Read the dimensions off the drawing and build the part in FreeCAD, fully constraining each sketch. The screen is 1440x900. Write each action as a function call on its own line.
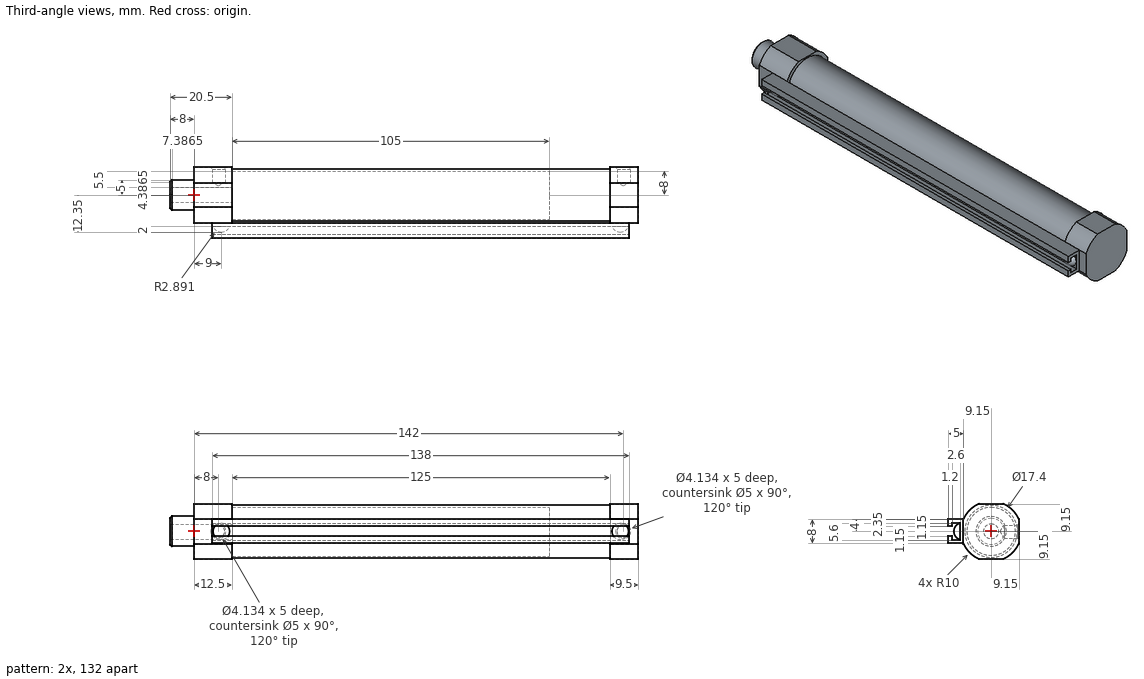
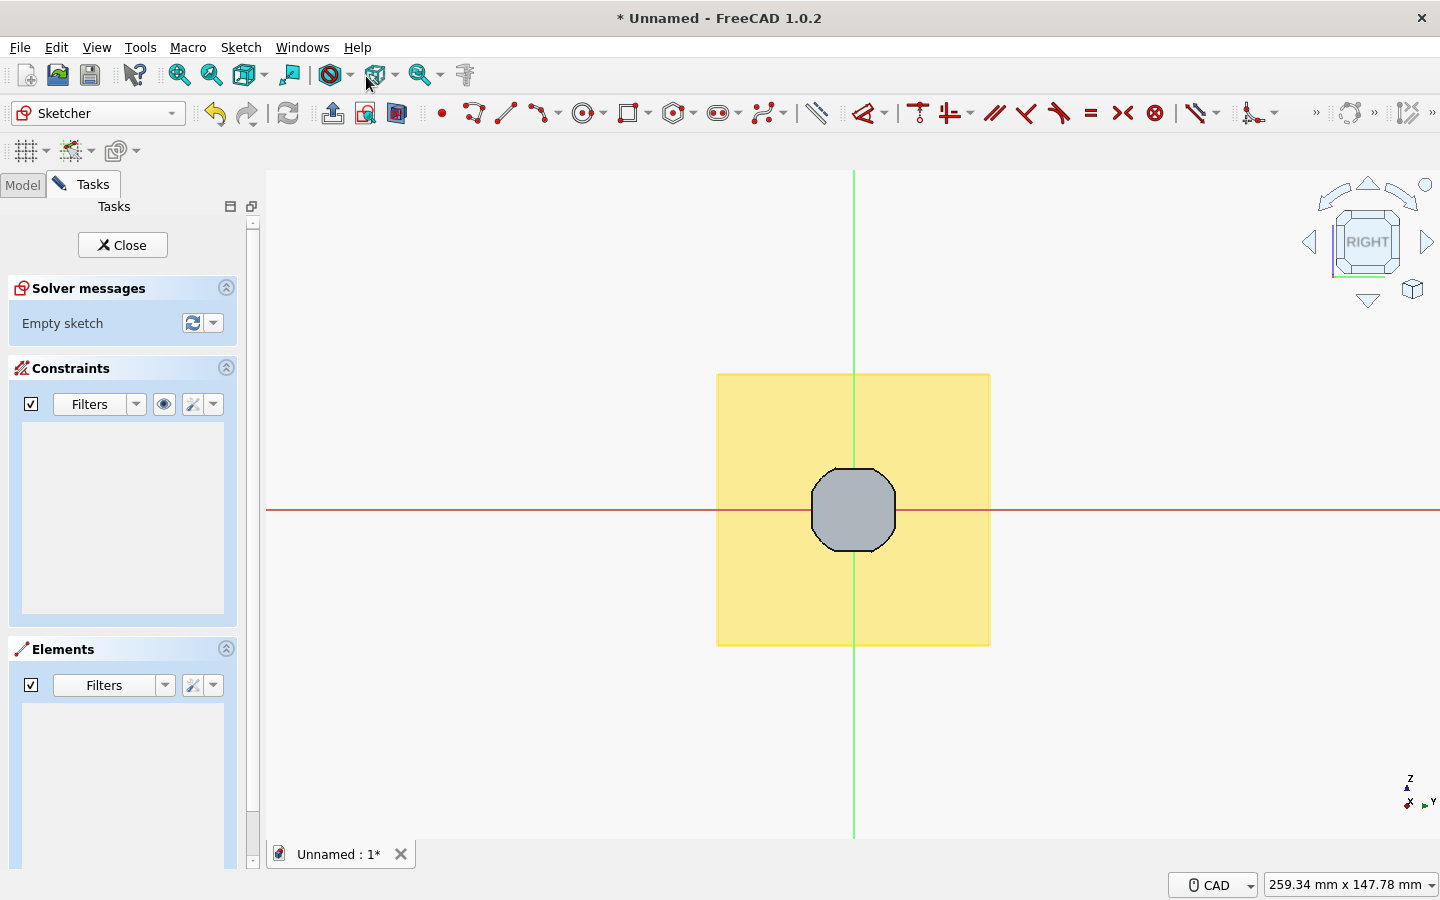
click(398, 114)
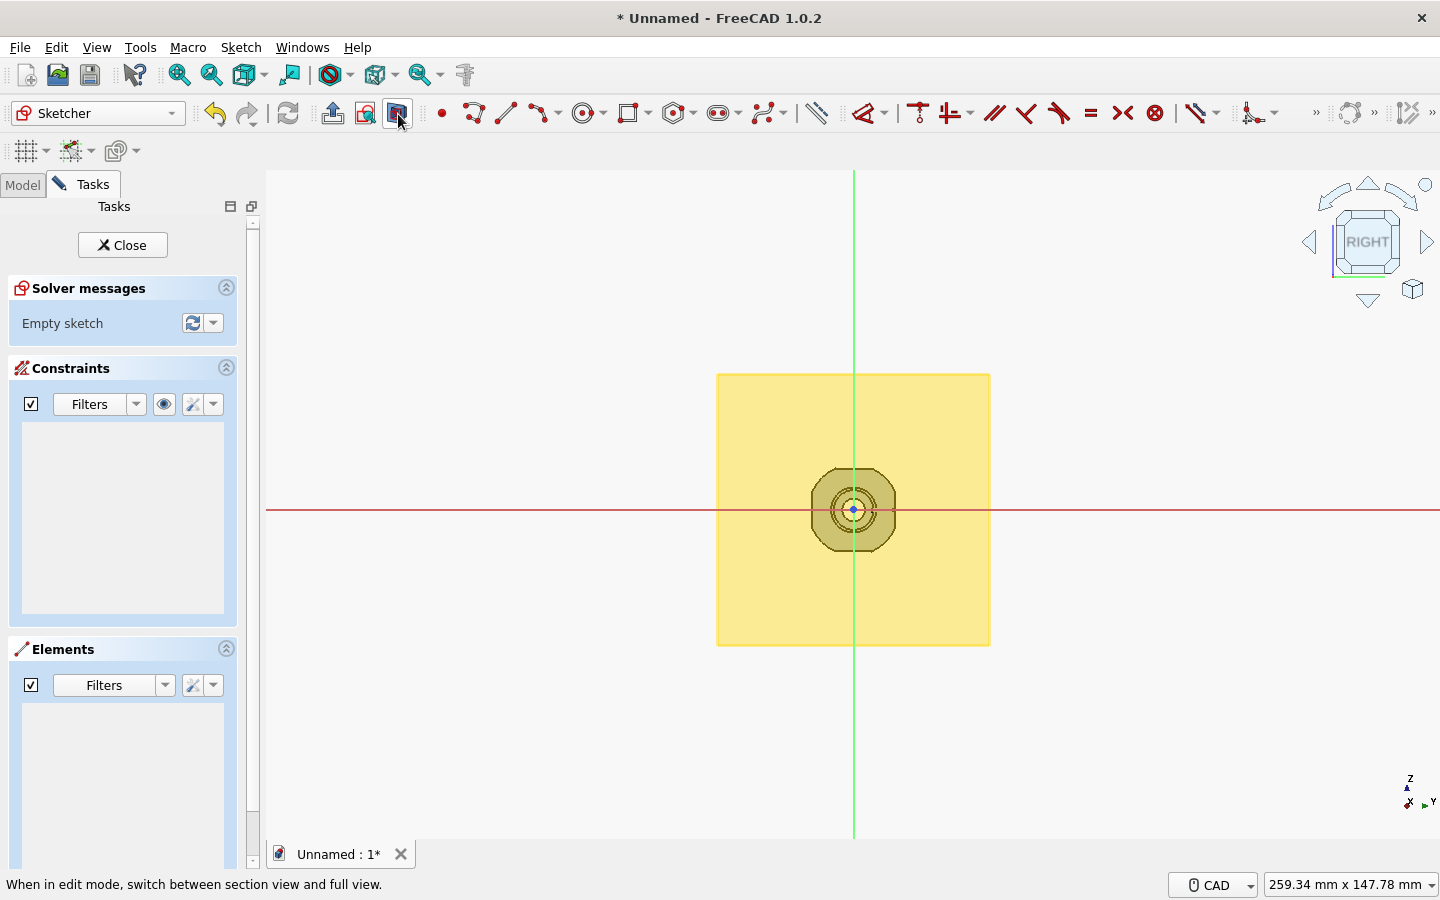
scroll(825, 511, up, 12)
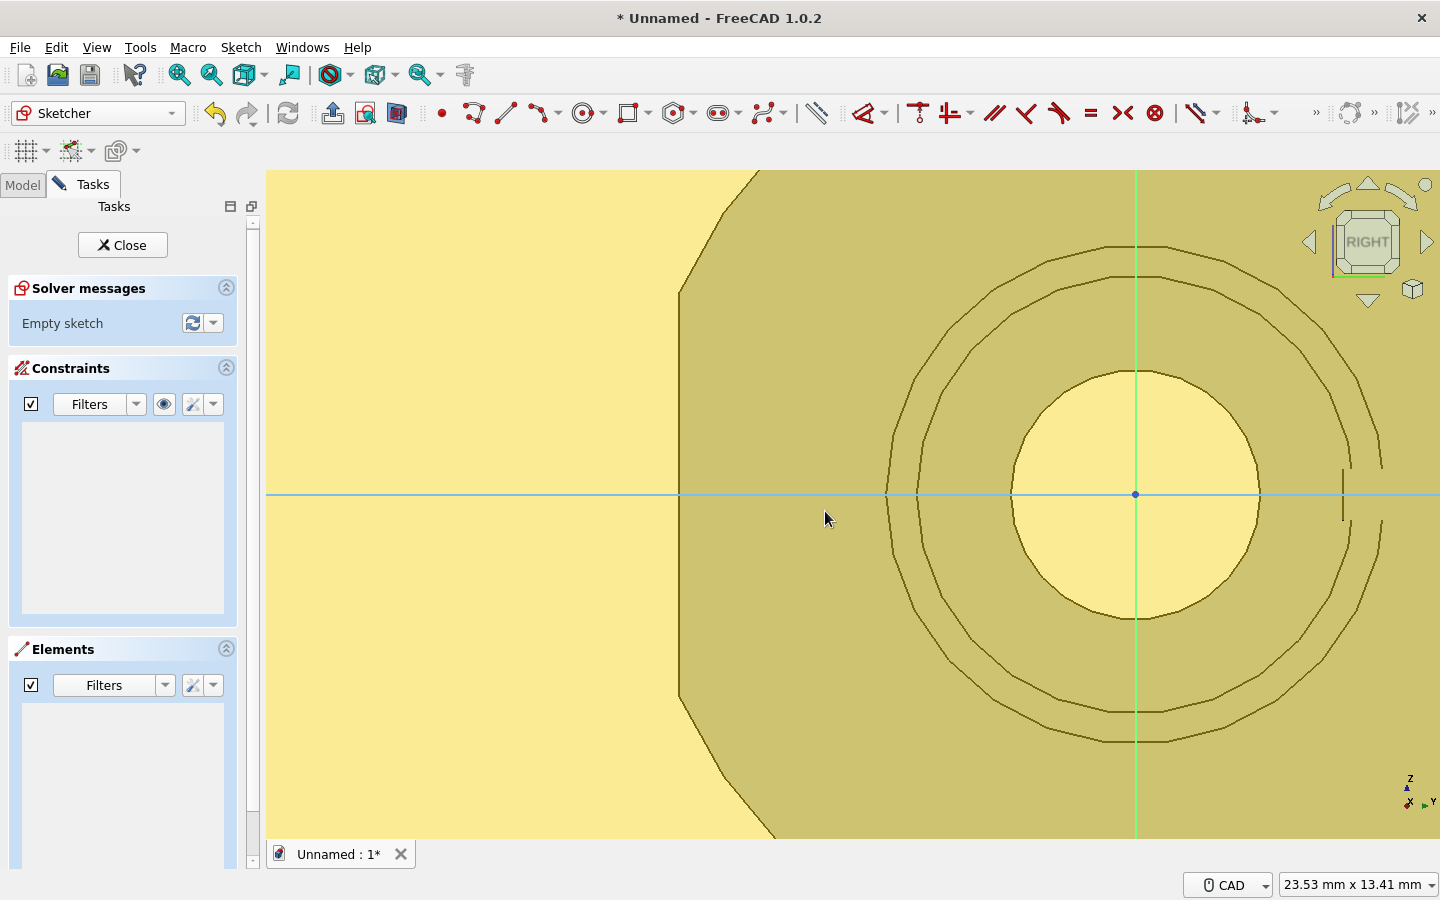
click(474, 114)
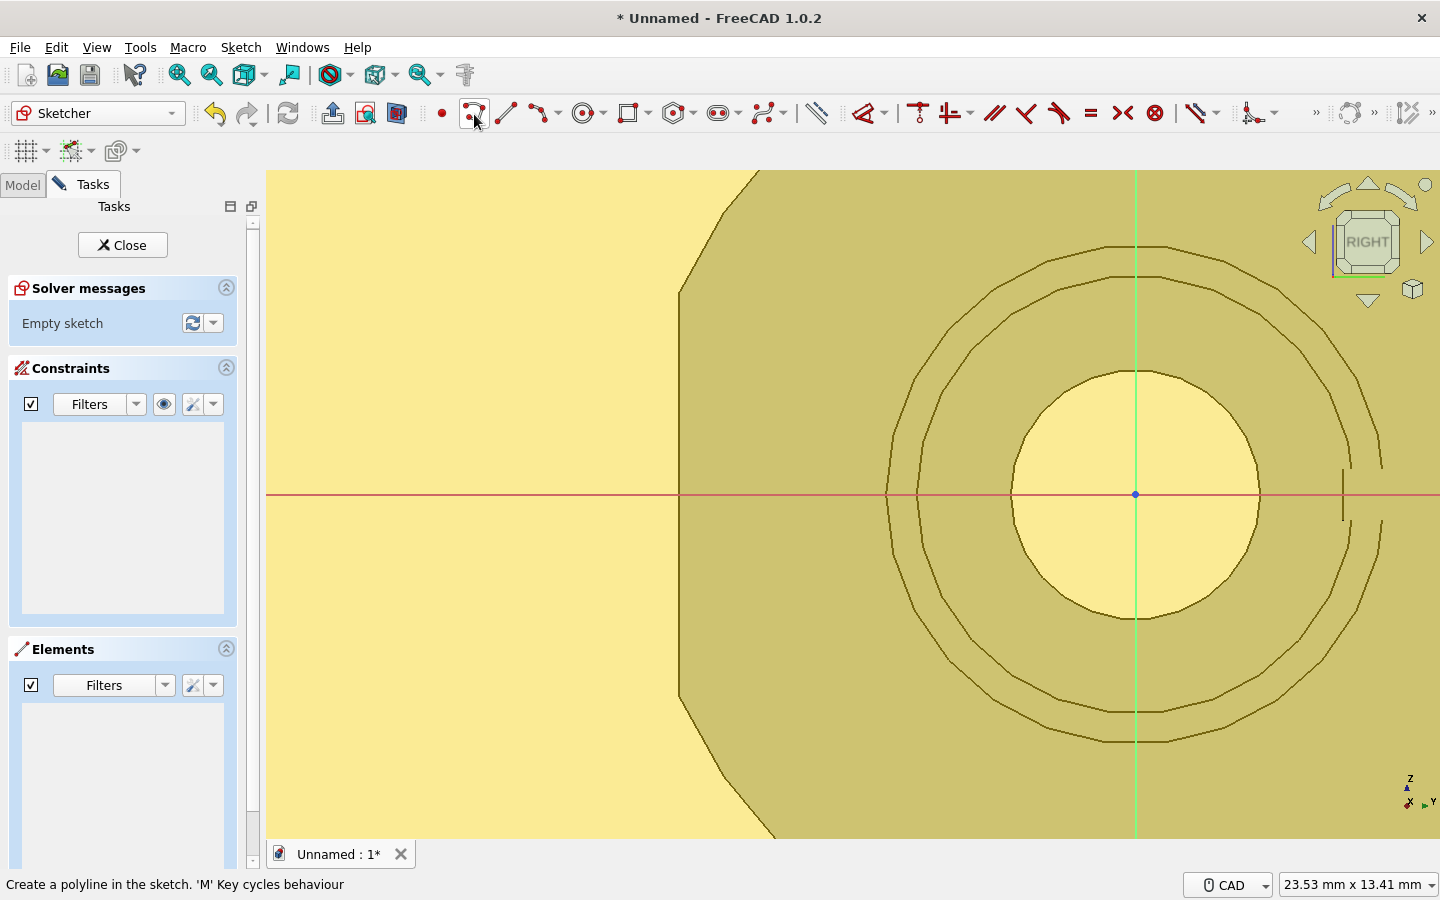
click(679, 295)
click(429, 295)
click(429, 412)
click(489, 412)
click(489, 355)
click(619, 355)
click(619, 634)
click(489, 634)
click(489, 577)
click(429, 577)
click(429, 694)
click(679, 694)
click(679, 296)
key(Escape)
key(Escape)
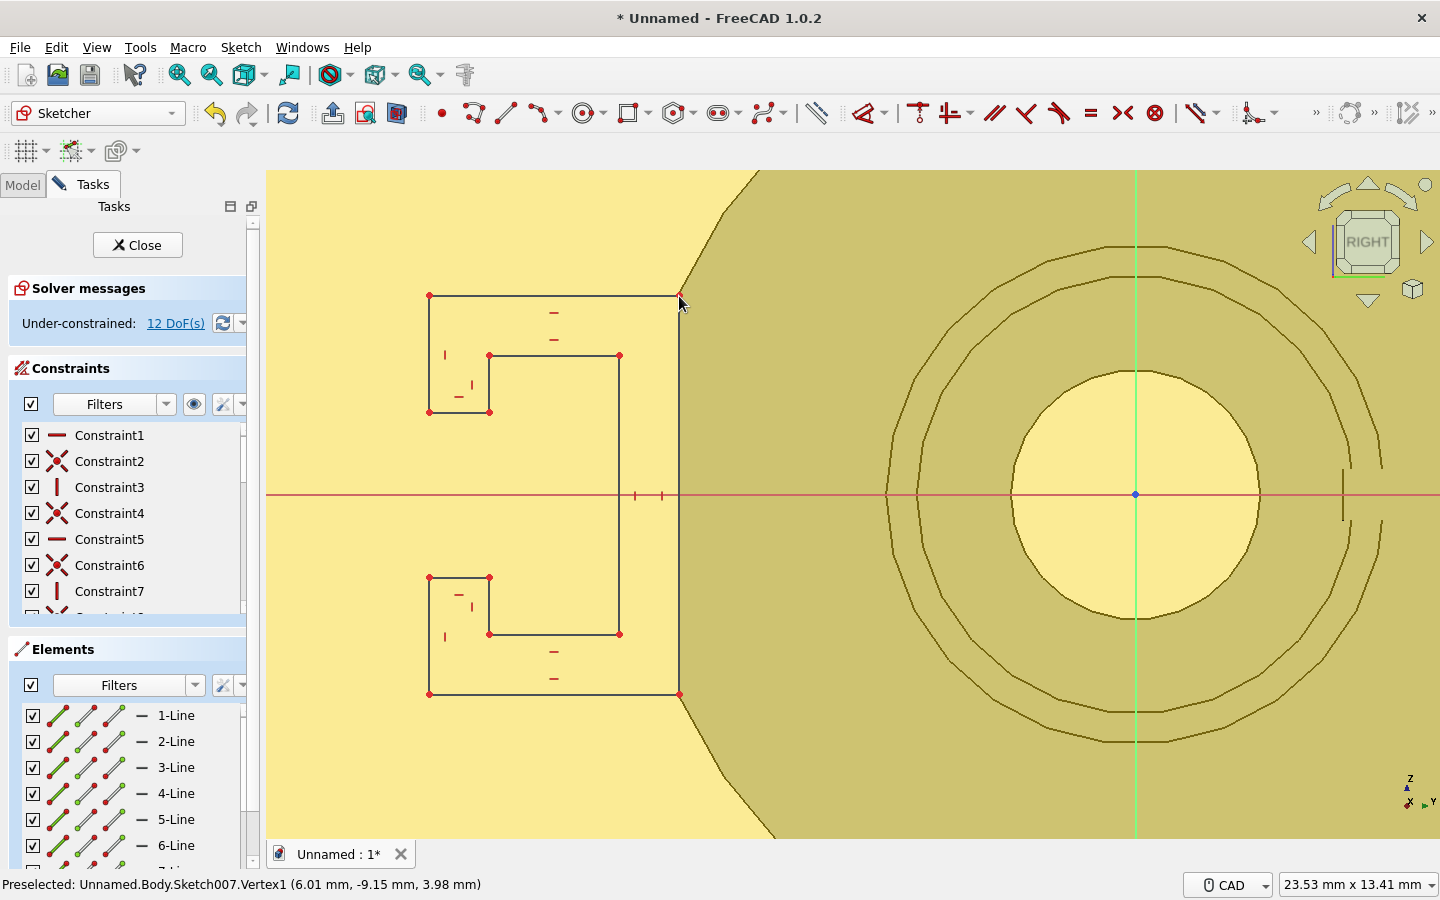
click(864, 114)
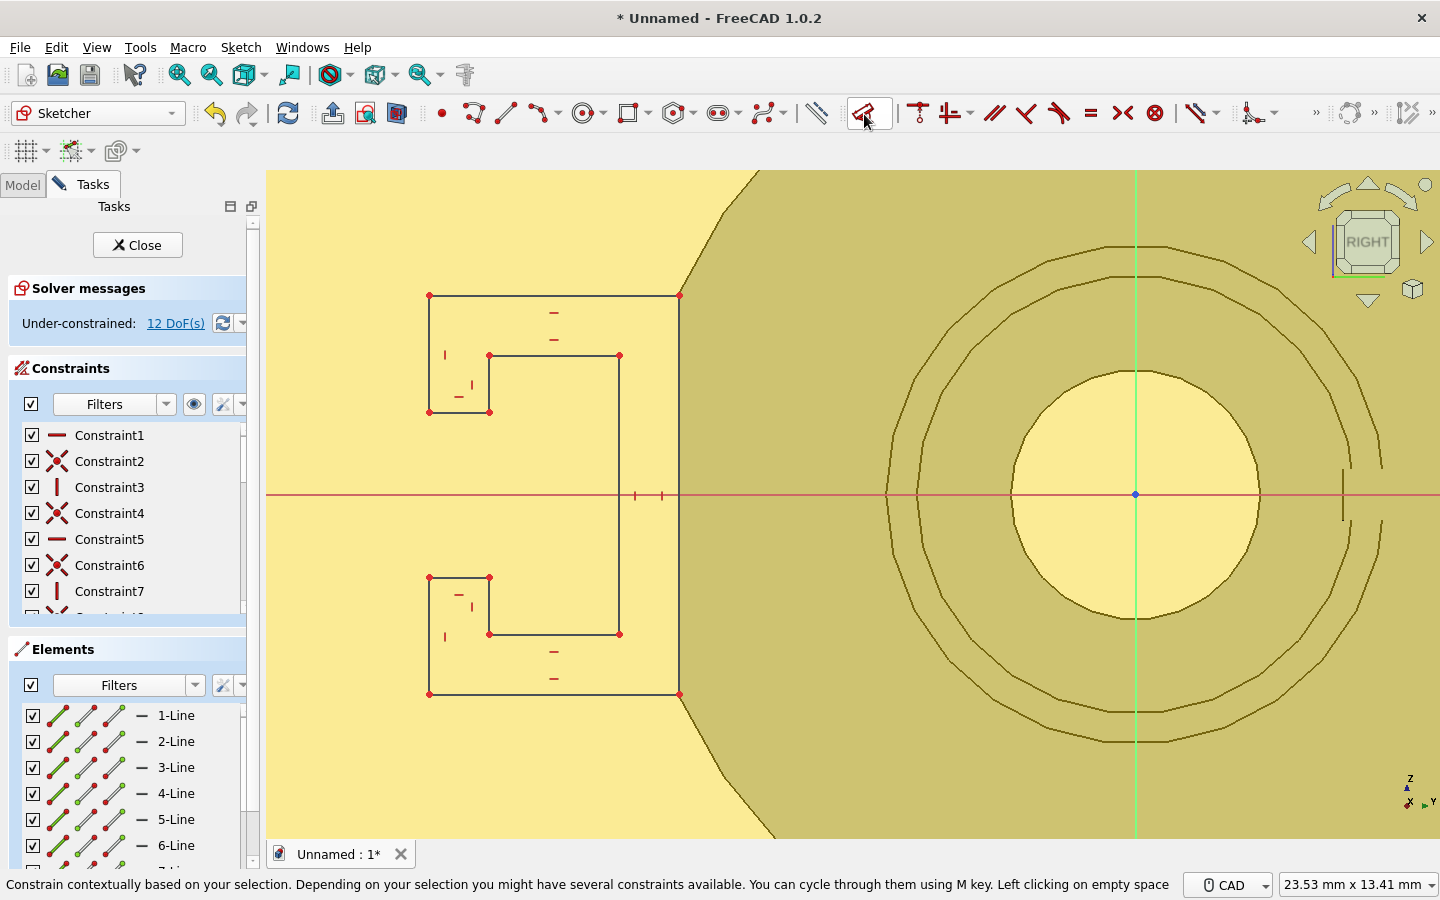
click(604, 296)
click(554, 262)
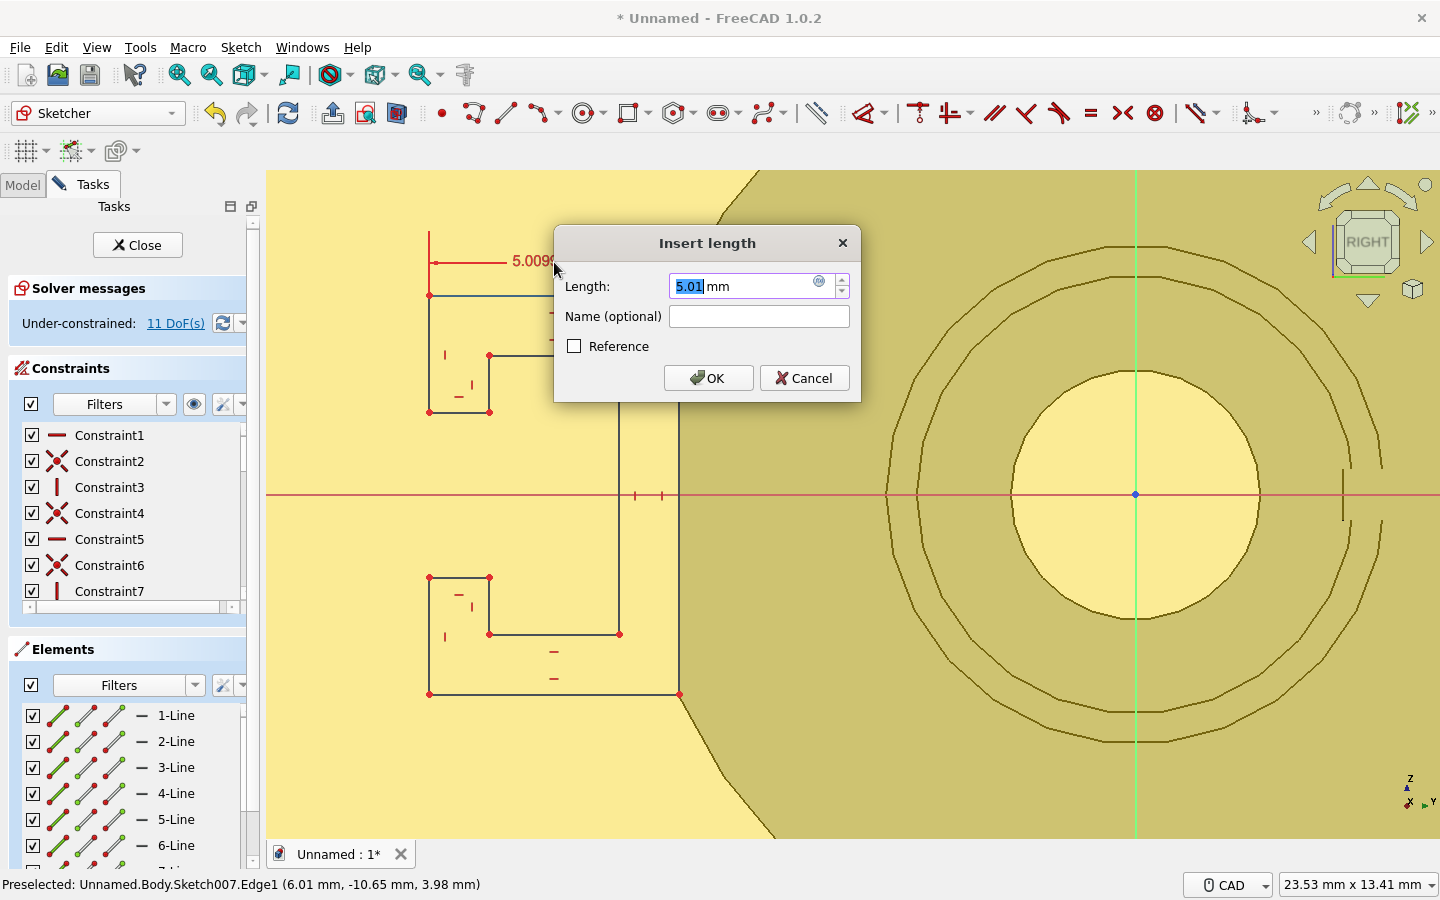
text(5)
key(Return)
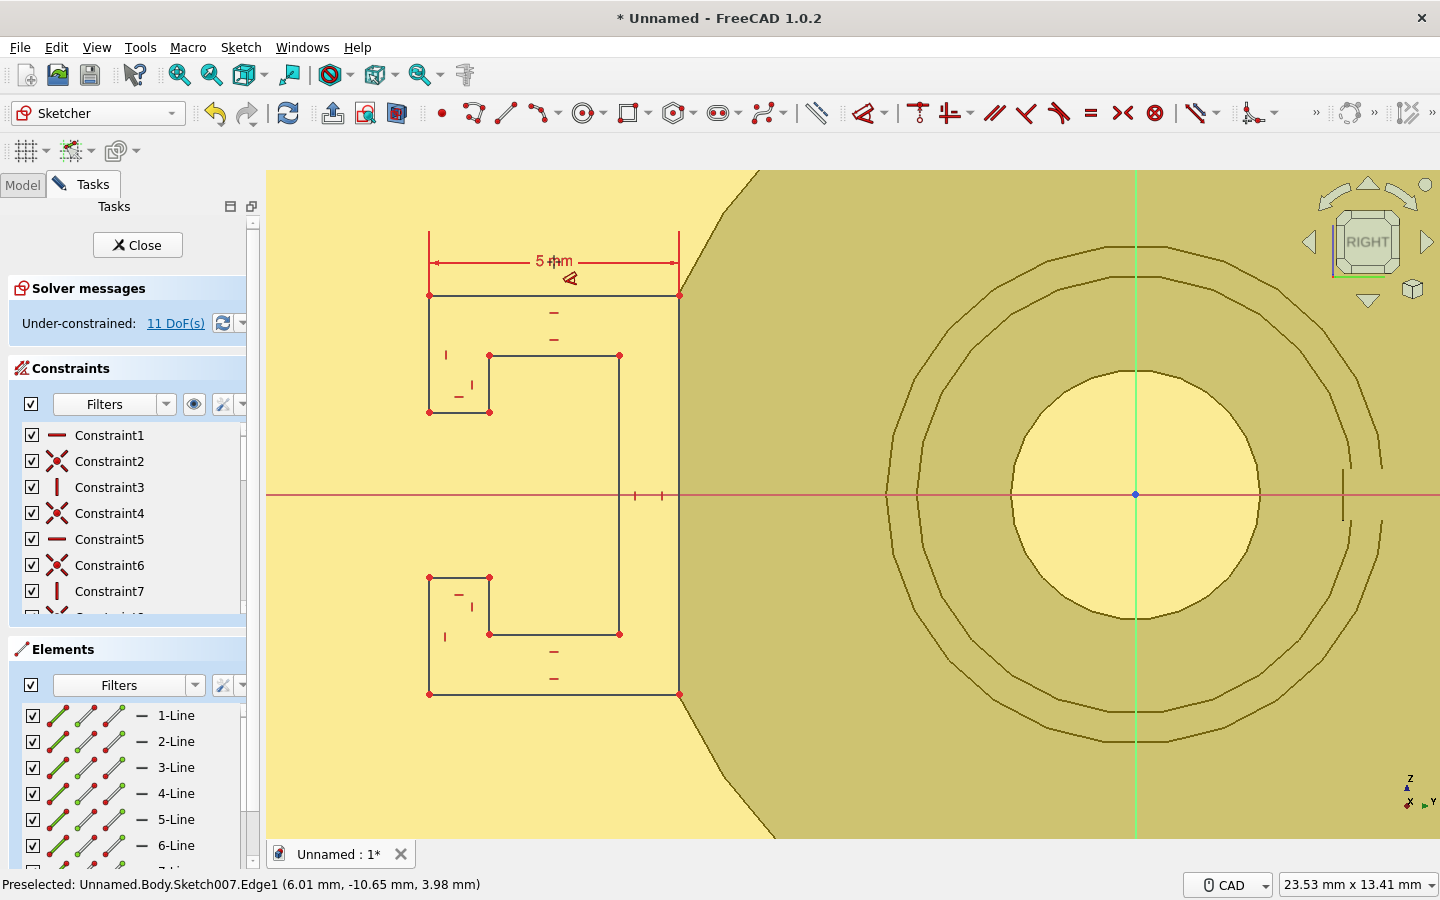
click(504, 695)
click(554, 729)